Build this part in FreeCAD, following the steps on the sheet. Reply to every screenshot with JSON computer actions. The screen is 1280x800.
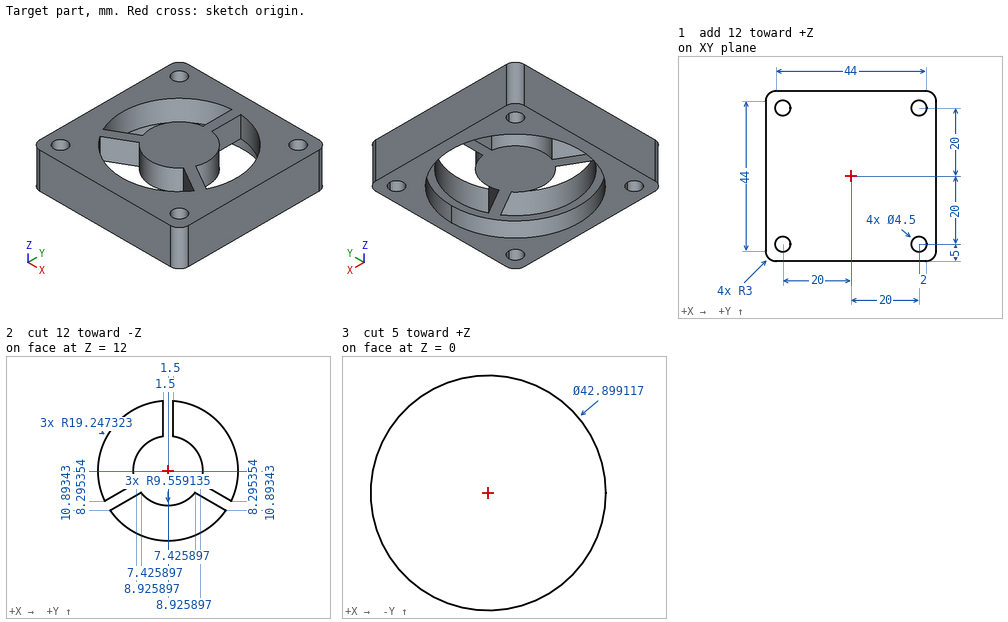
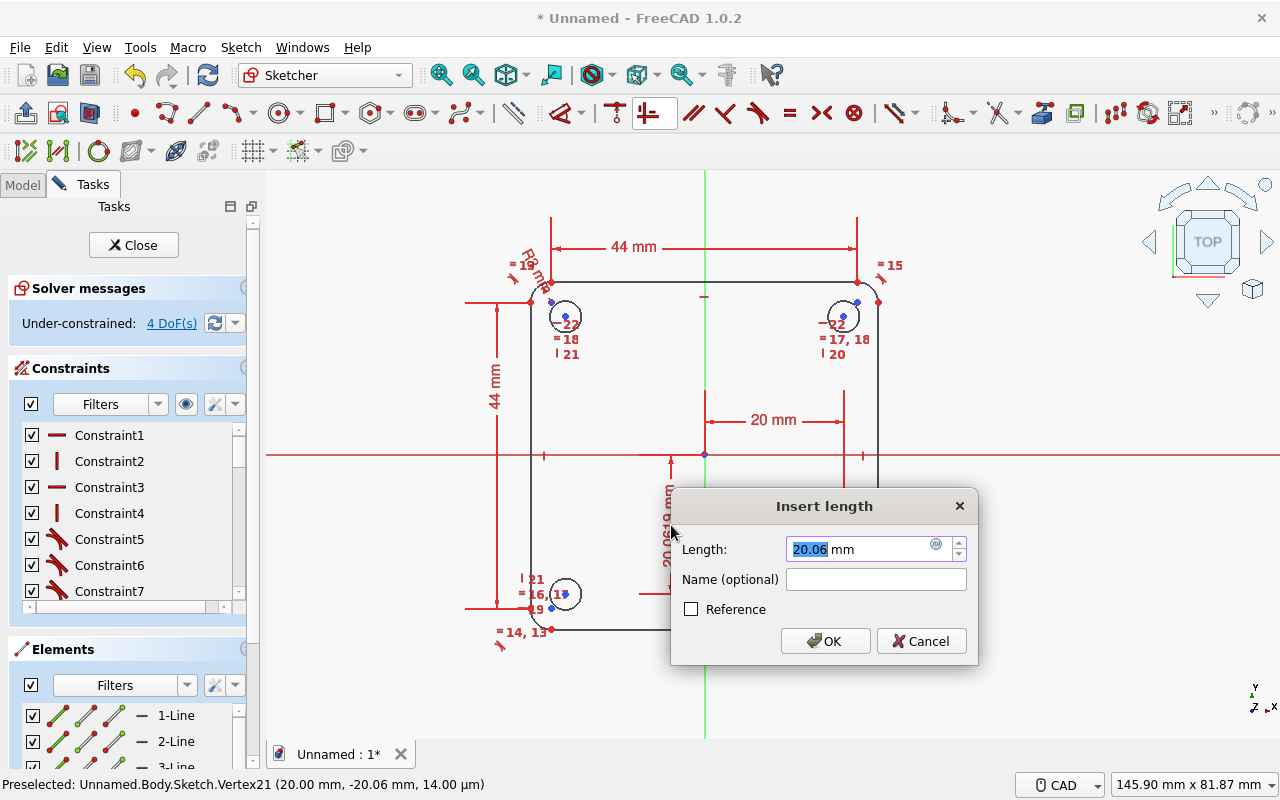
{"action": "type", "text": "20"}
{"action": "key", "text": "Return"}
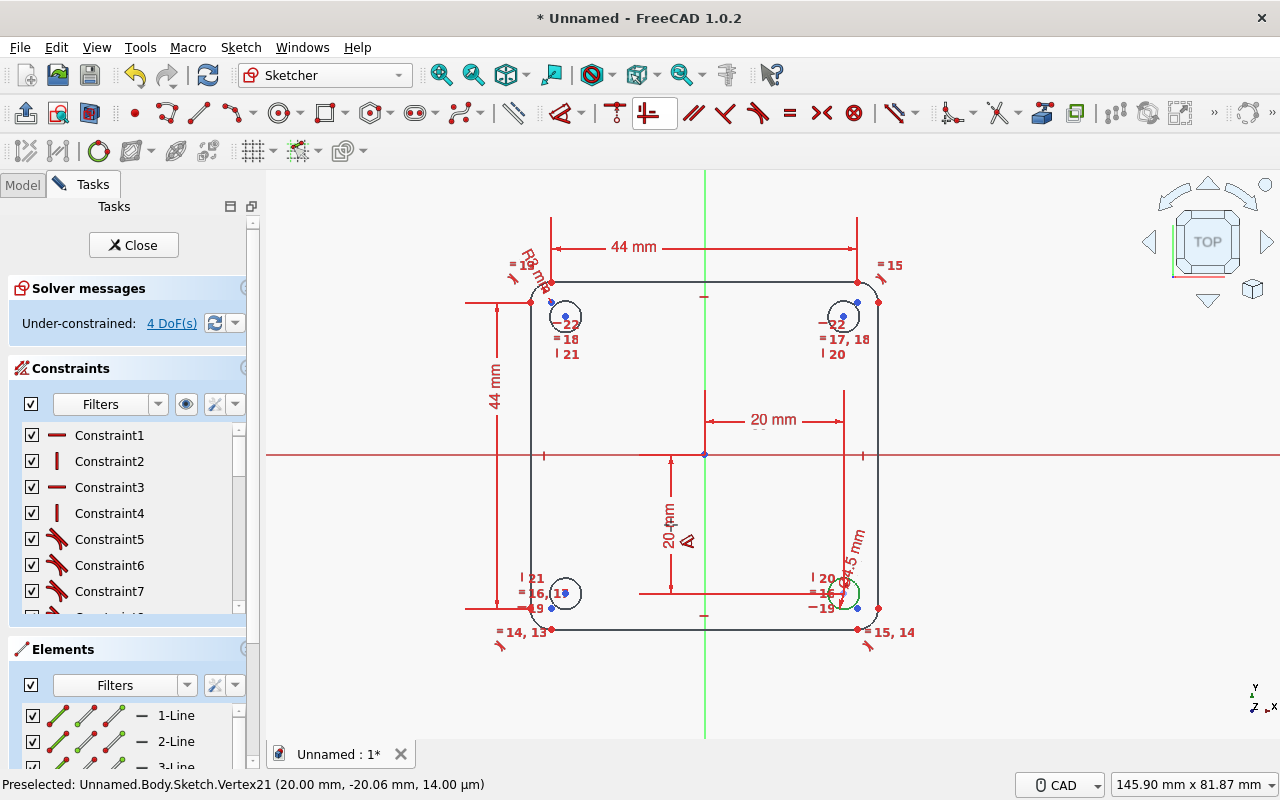
{"action": "left_click", "coordinate": [566, 594]}
{"action": "left_click", "coordinate": [635, 421]}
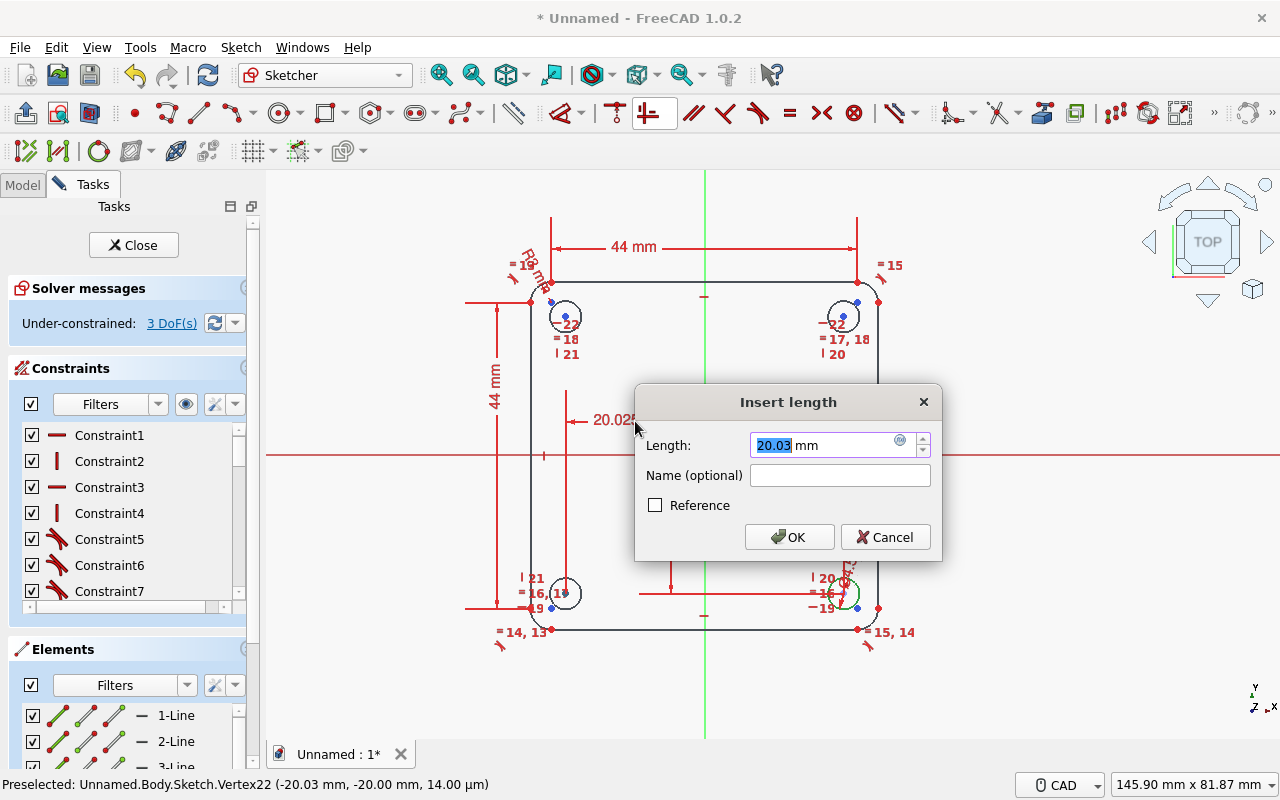
{"action": "type", "text": "20"}
{"action": "key", "text": "Return"}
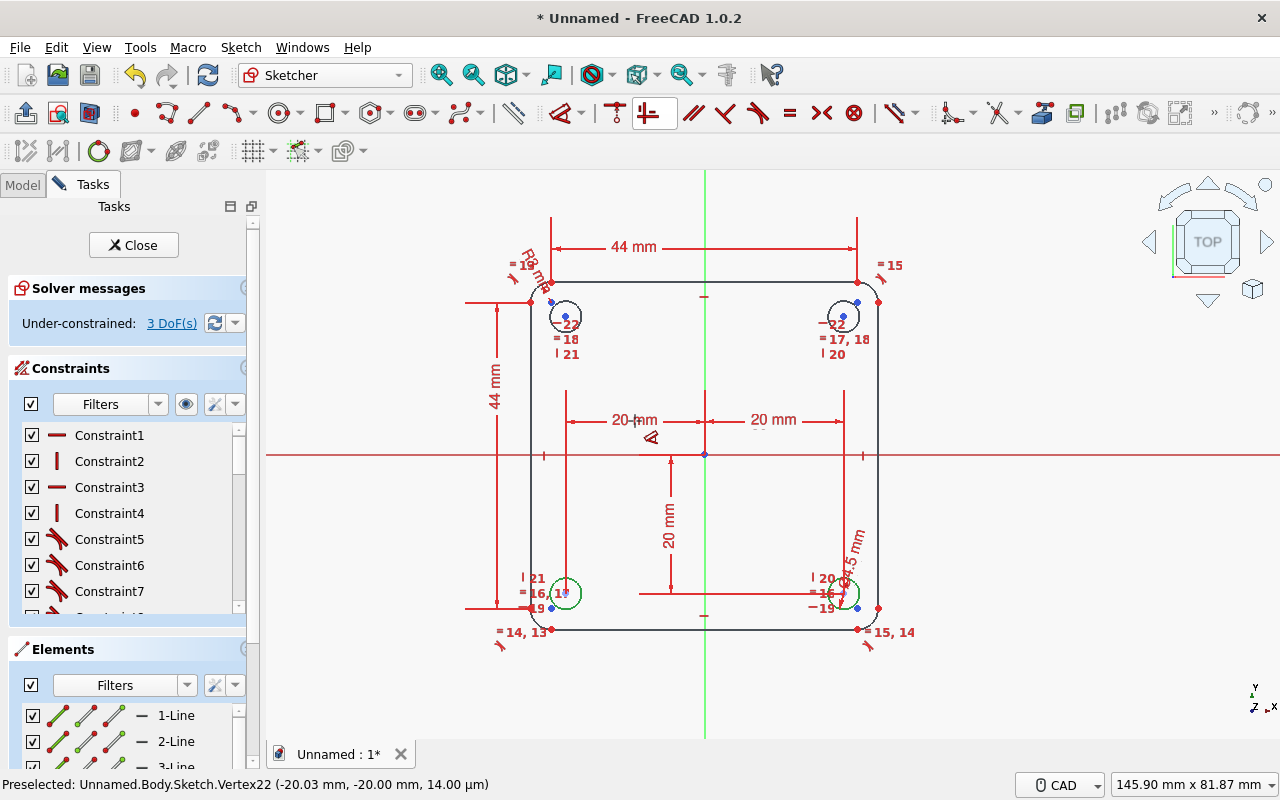
{"action": "left_click", "coordinate": [844, 317]}
{"action": "left_click", "coordinate": [671, 386]}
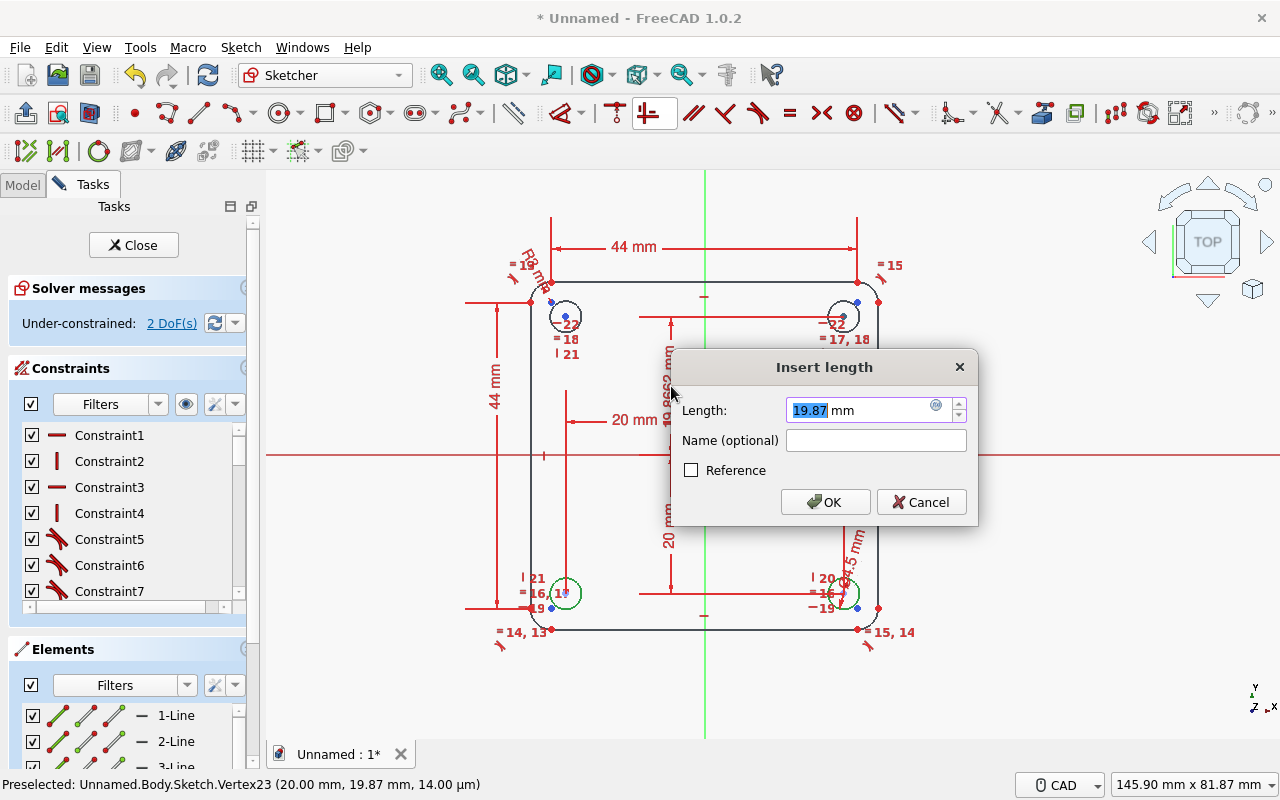
{"action": "type", "text": "20"}
{"action": "key", "text": "Return"}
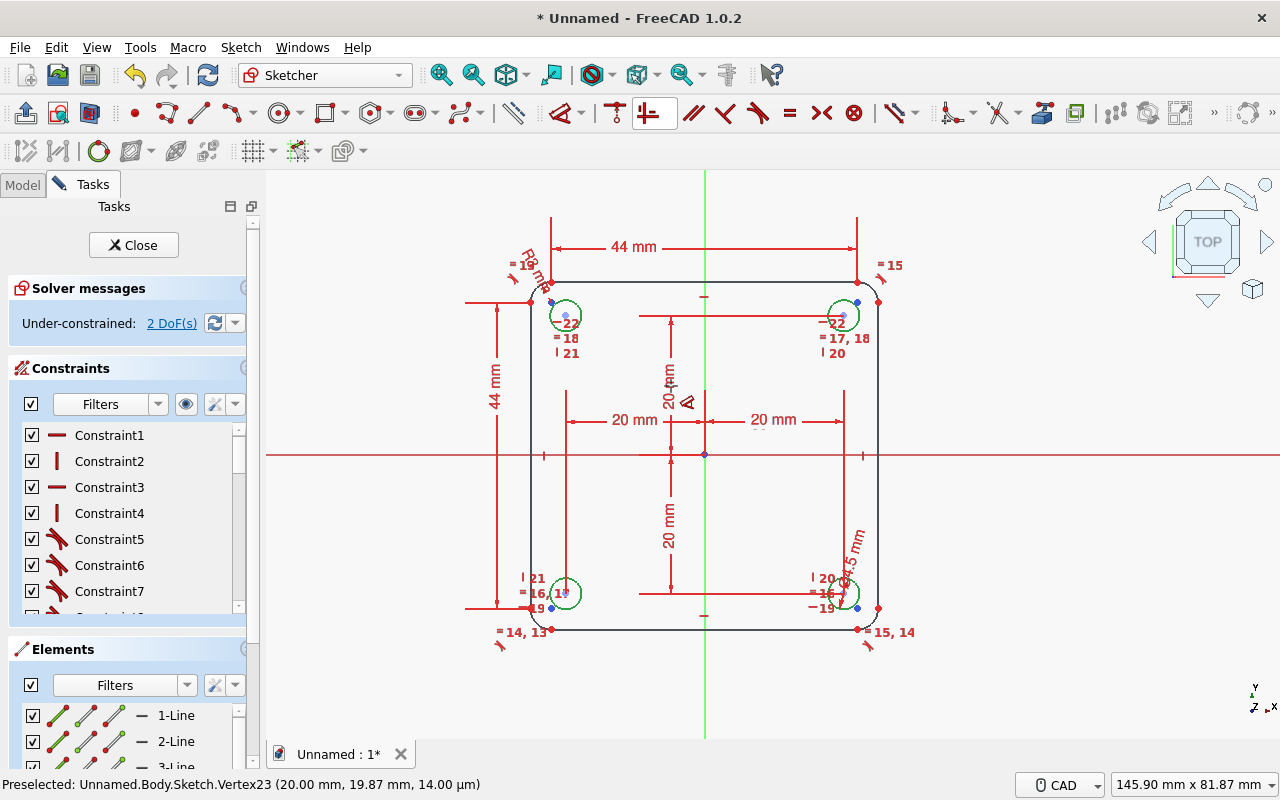
{"action": "scroll", "coordinate": [857, 630], "scroll_direction": "up", "scroll_amount": 6}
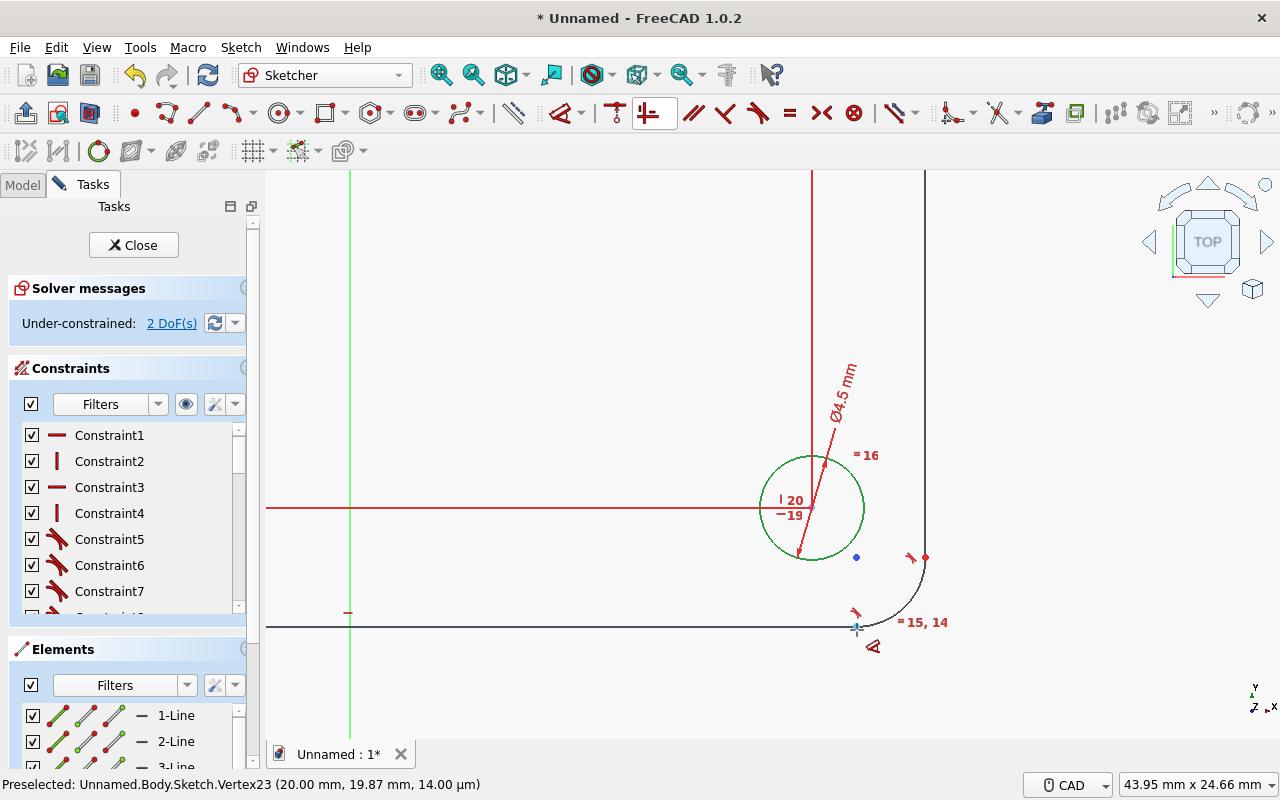
{"action": "left_click", "coordinate": [856, 627]}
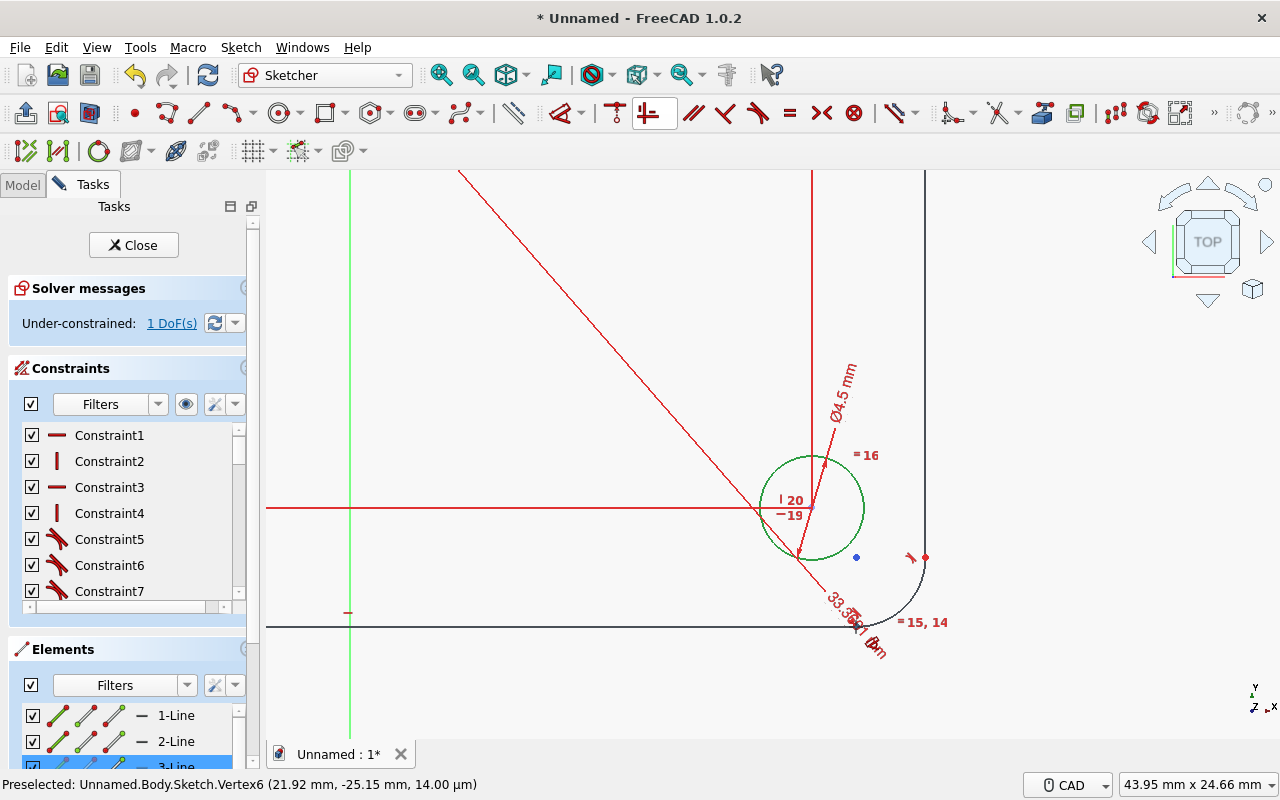
{"action": "left_click", "coordinate": [812, 508]}
{"action": "left_click", "coordinate": [834, 661]}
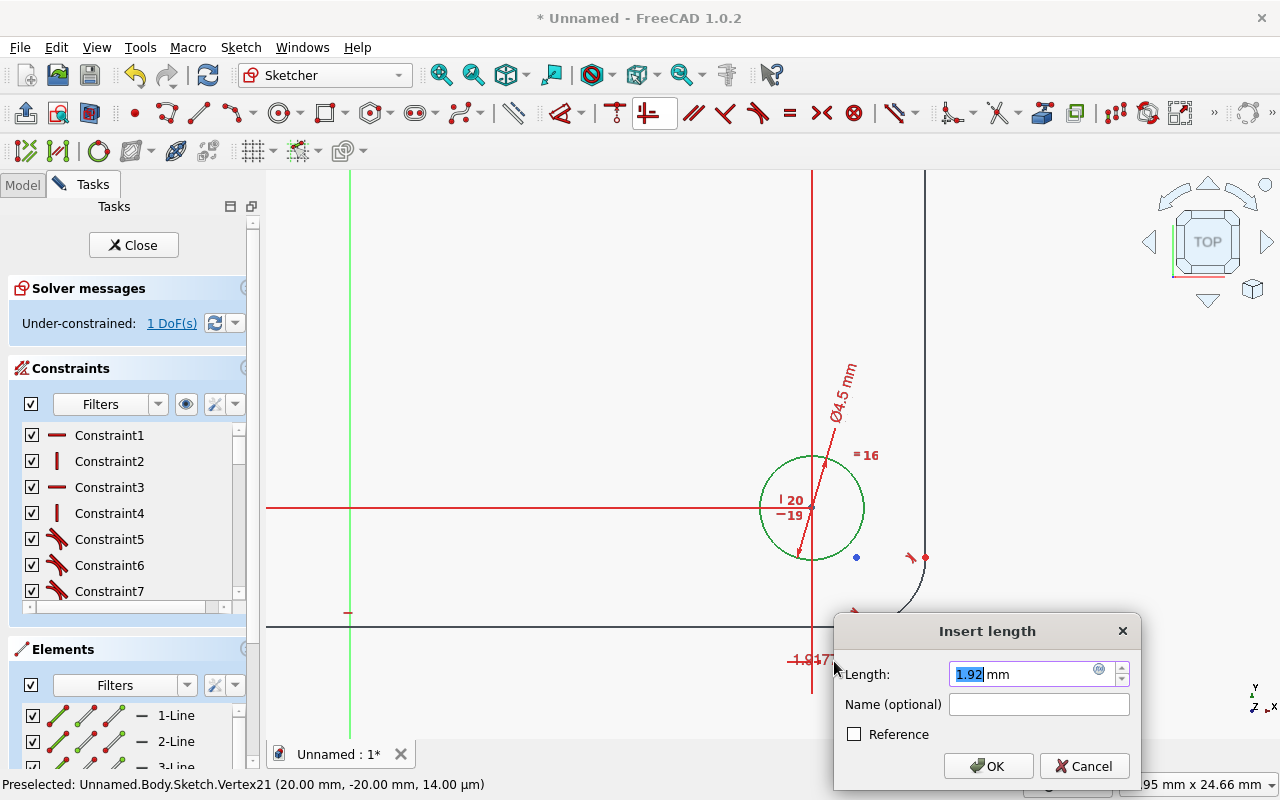
{"action": "type", "text": "2"}
{"action": "key", "text": "Return"}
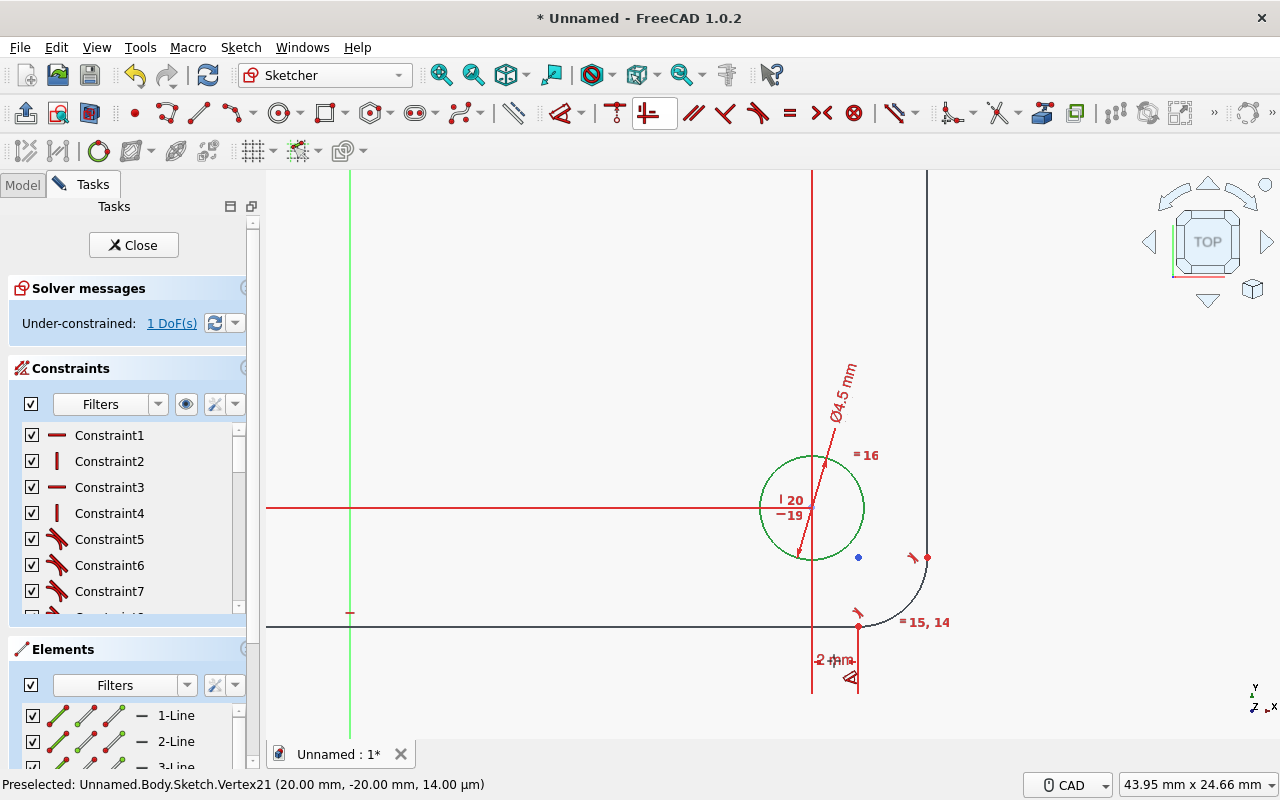
{"action": "scroll", "coordinate": [857, 630], "scroll_direction": "down", "scroll_amount": 6}